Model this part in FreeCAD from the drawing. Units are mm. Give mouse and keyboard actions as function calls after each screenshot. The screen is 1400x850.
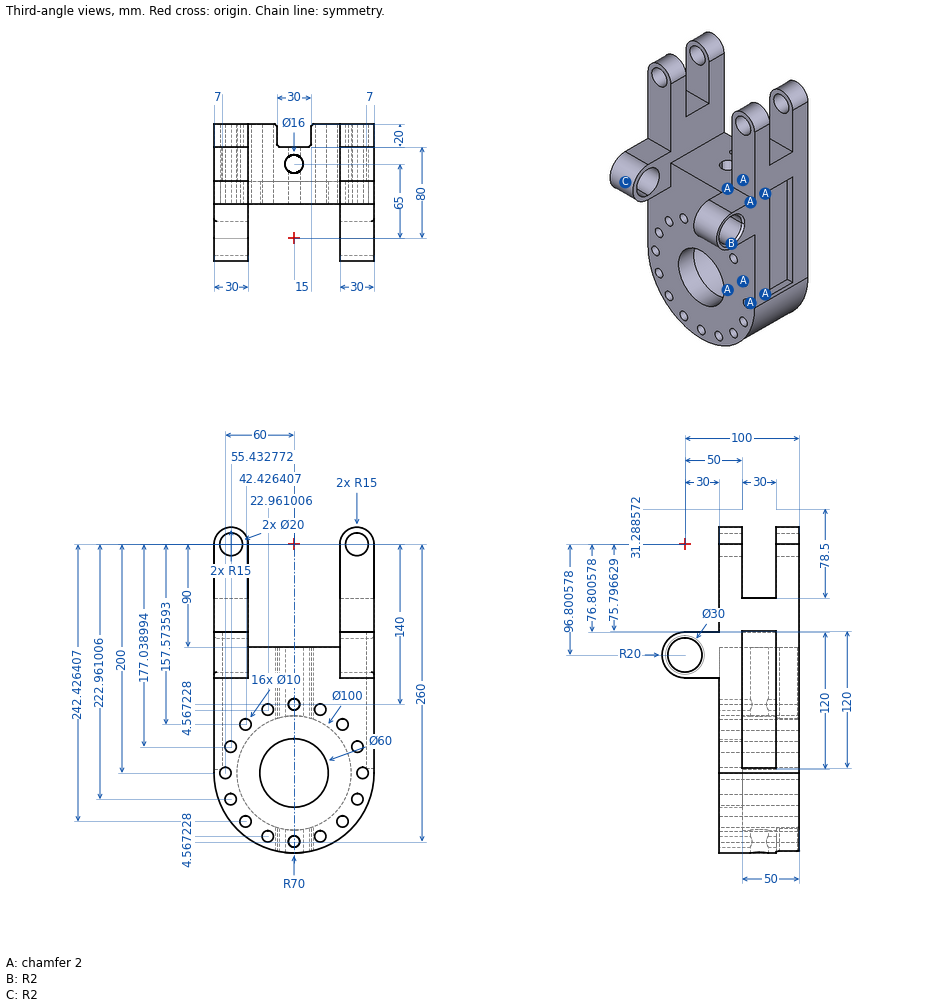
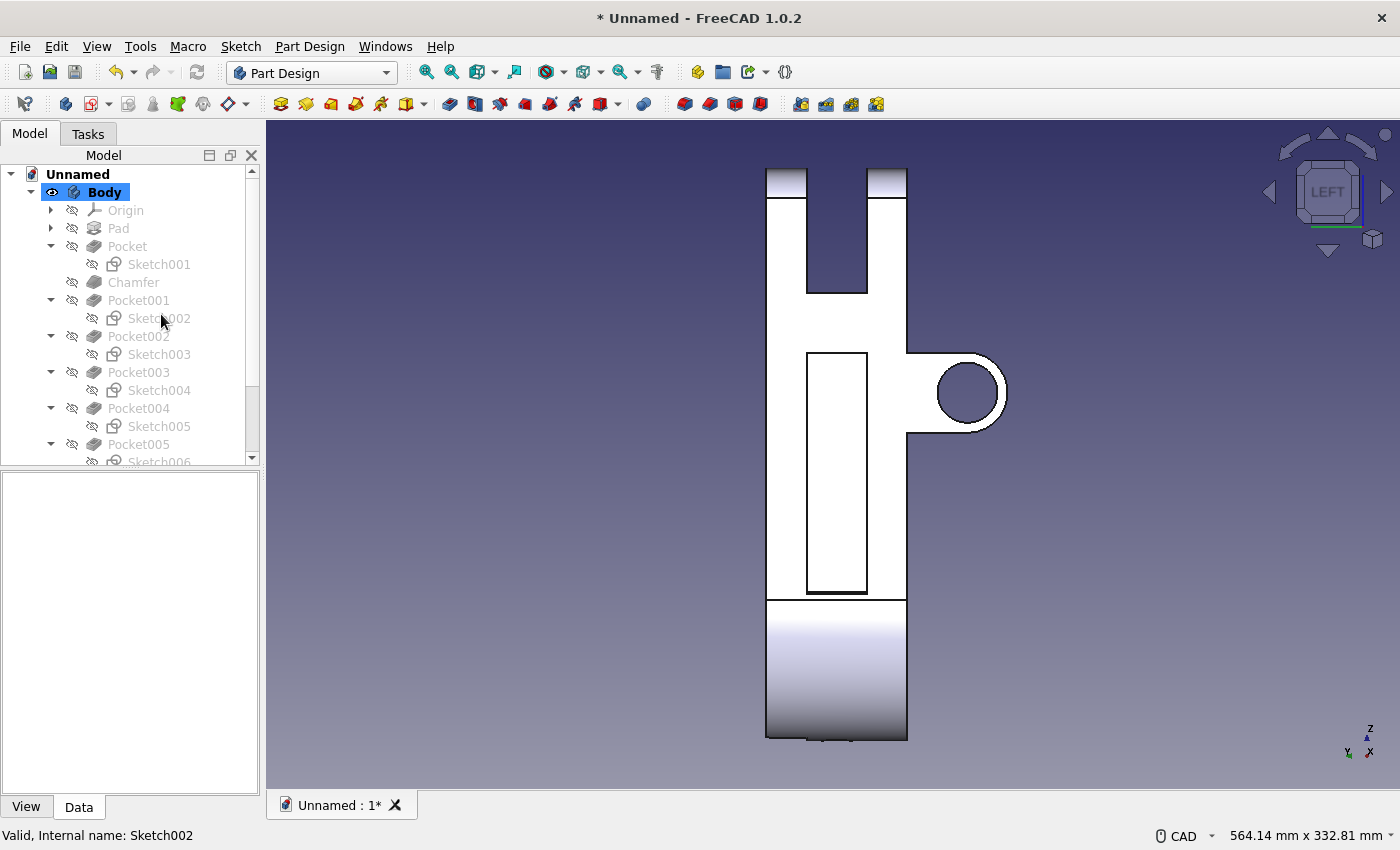
click(51, 210)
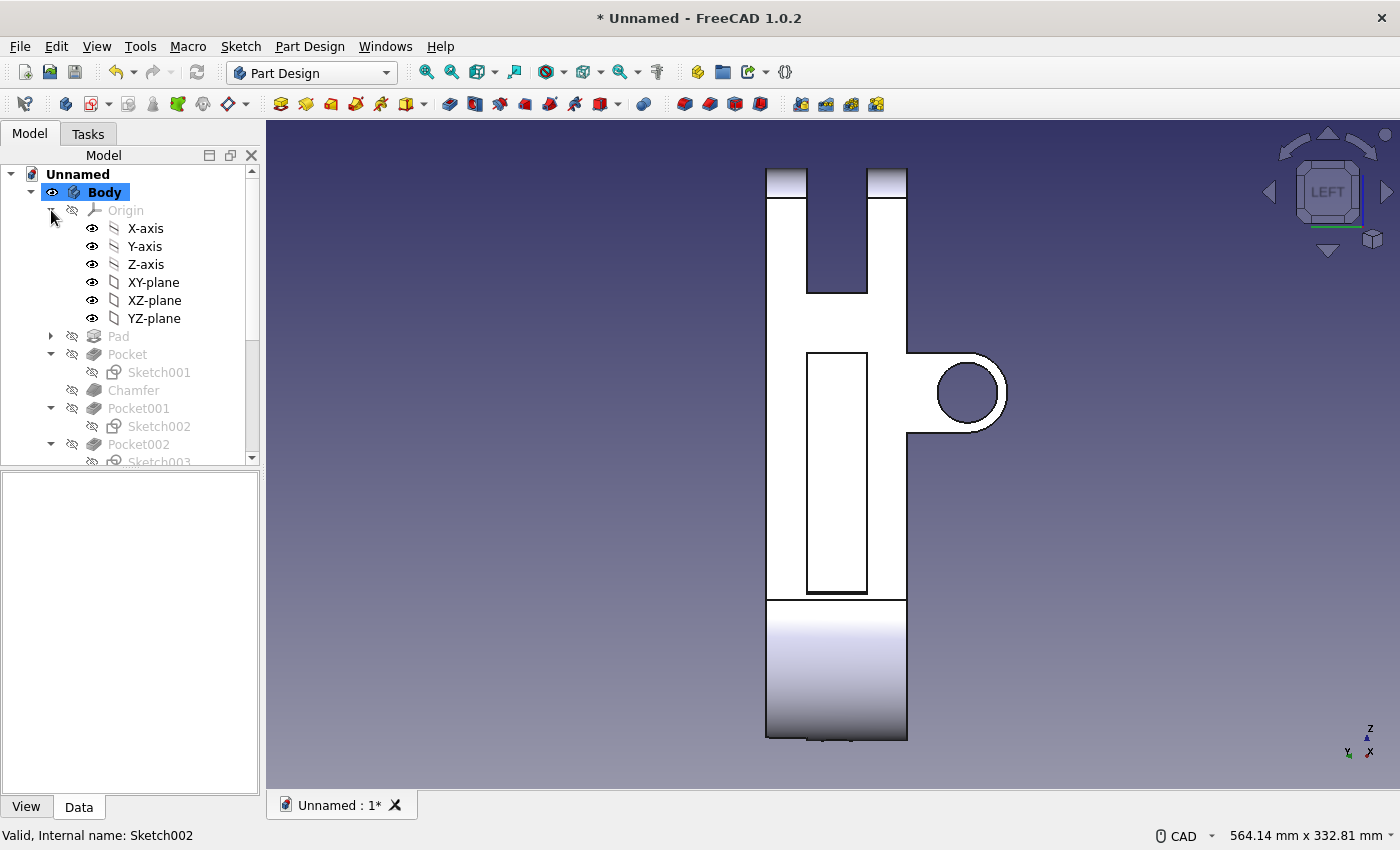
click(137, 318)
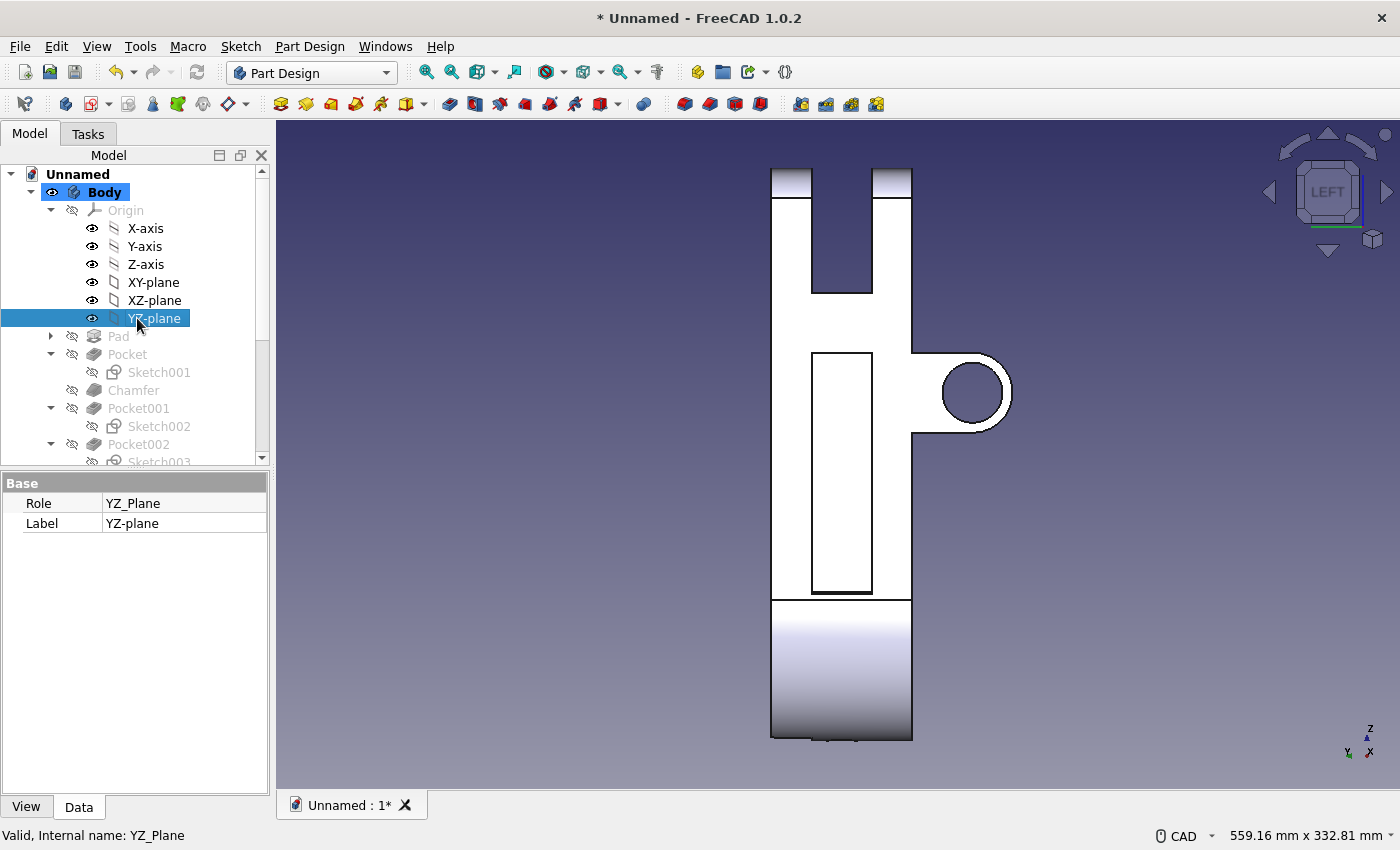
click(228, 104)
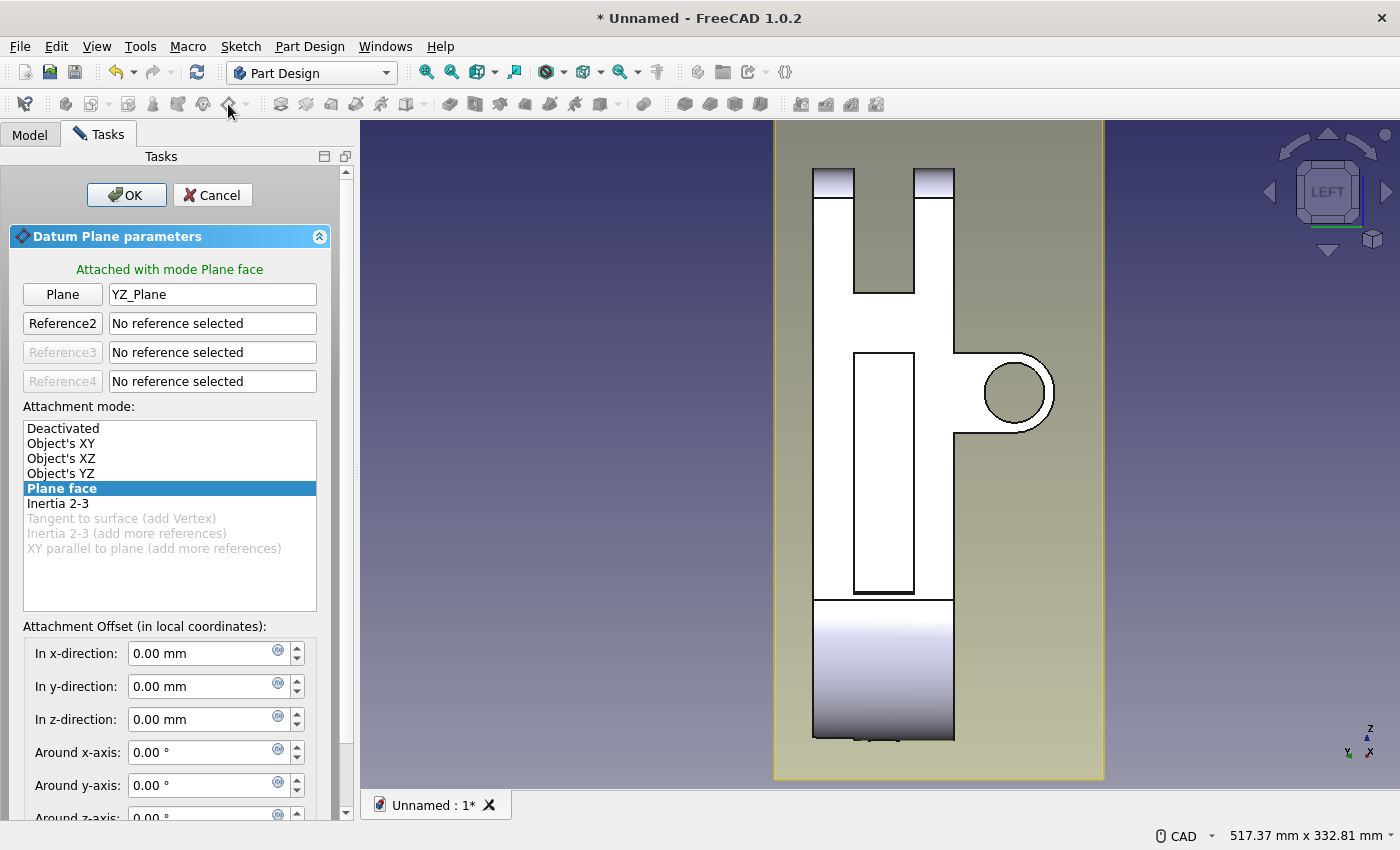
triple_click(210, 720)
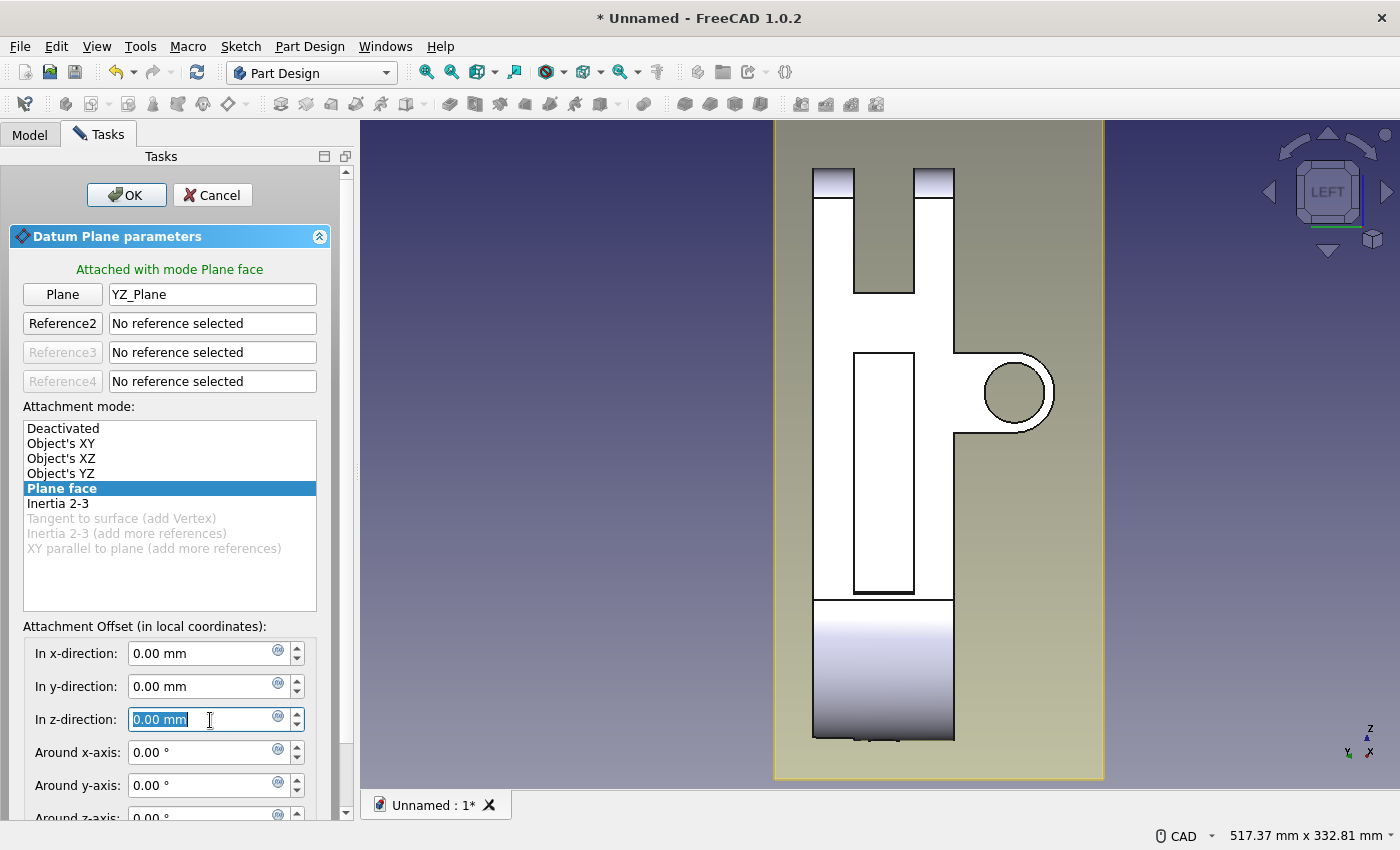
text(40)
key(Tab)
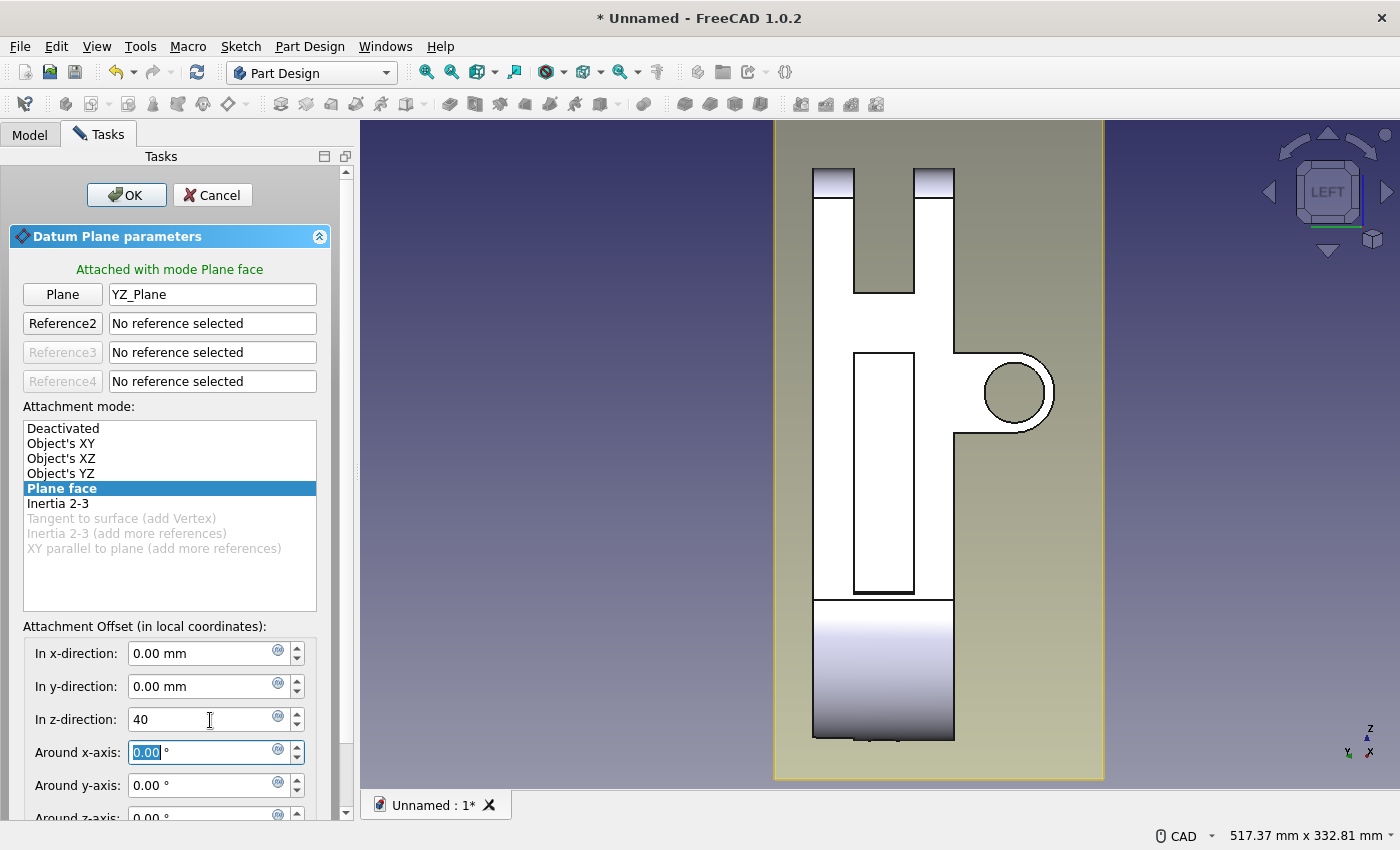
click(127, 195)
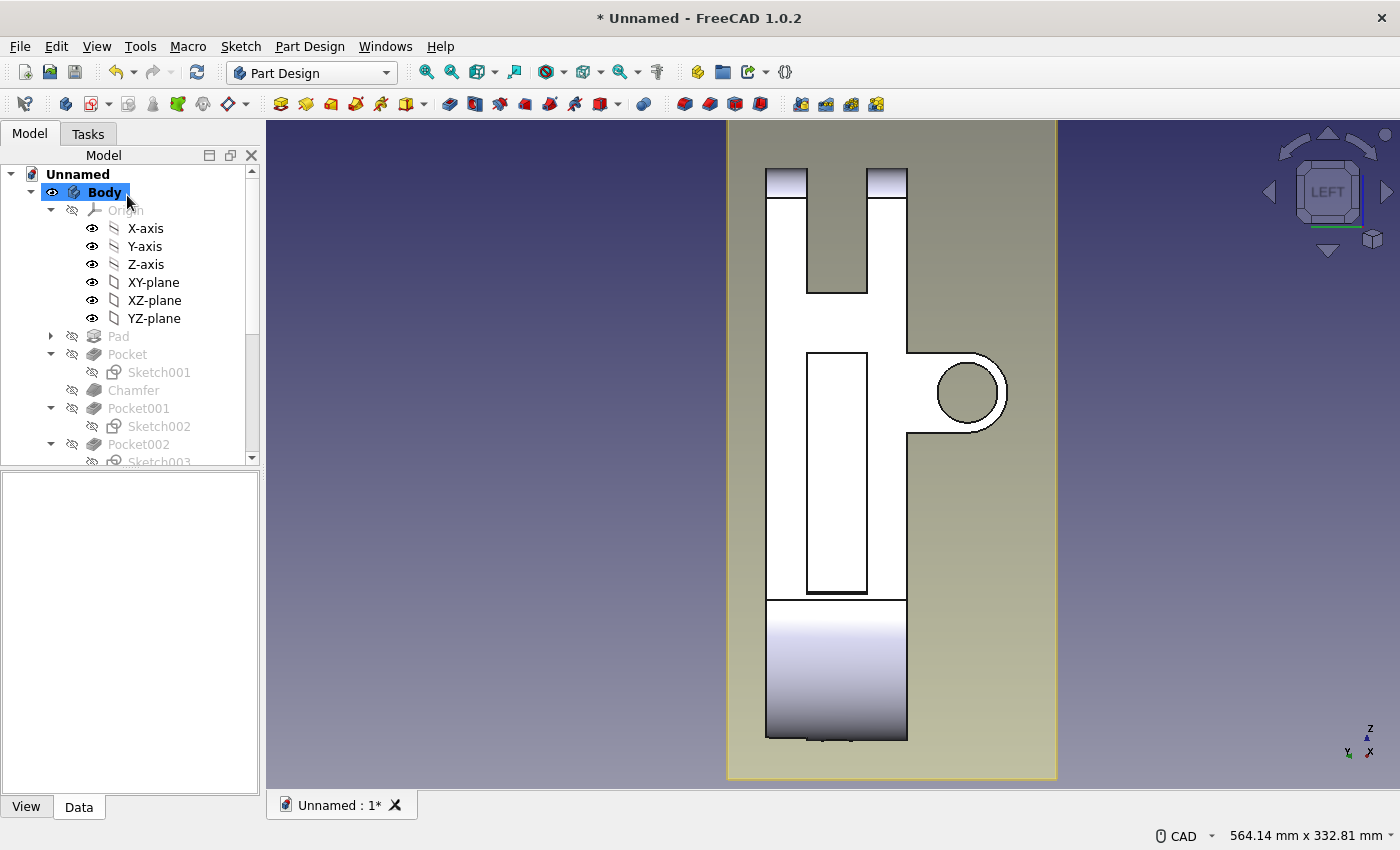
scroll(101, 314, down, 3)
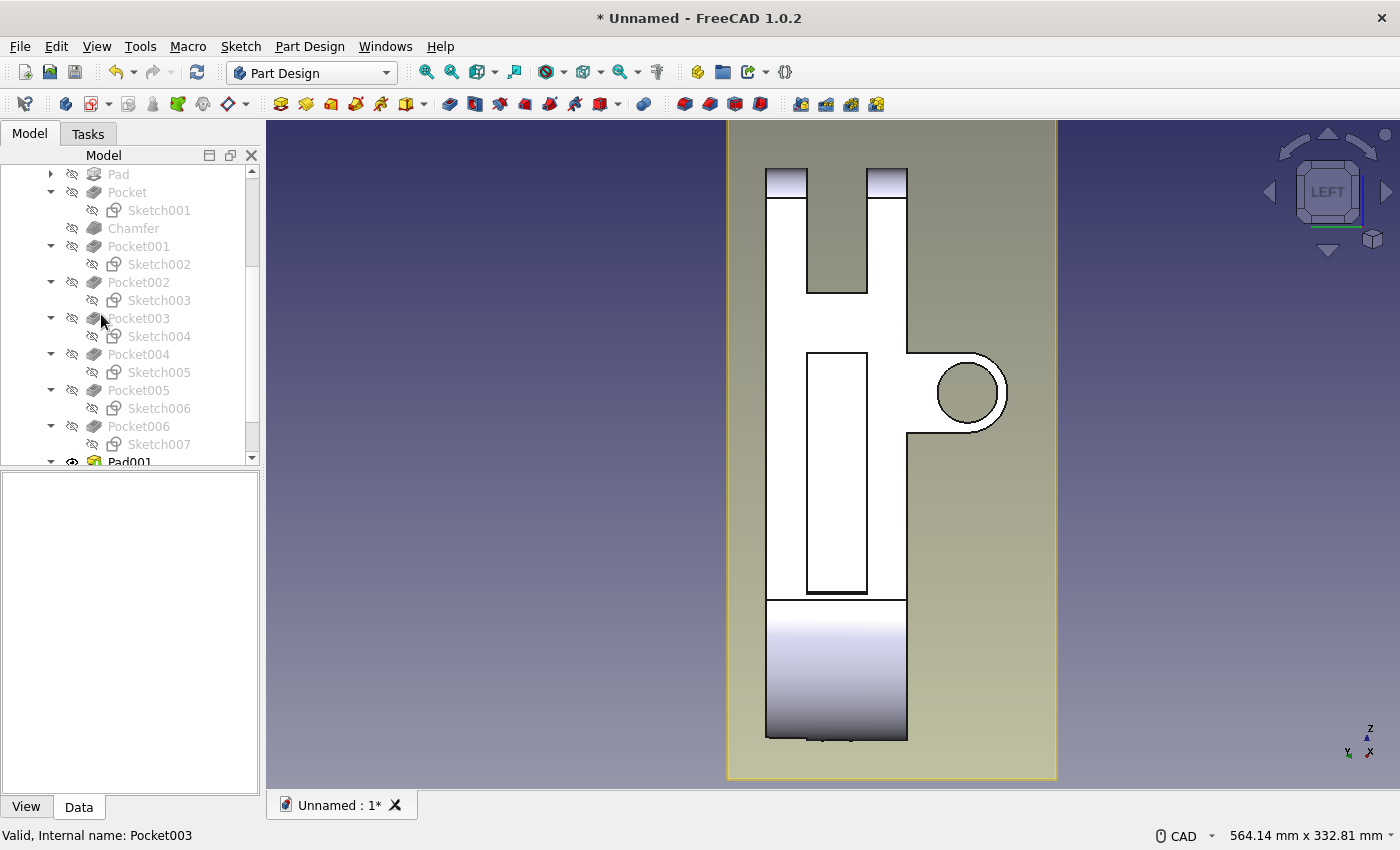
scroll(141, 314, up, 15)